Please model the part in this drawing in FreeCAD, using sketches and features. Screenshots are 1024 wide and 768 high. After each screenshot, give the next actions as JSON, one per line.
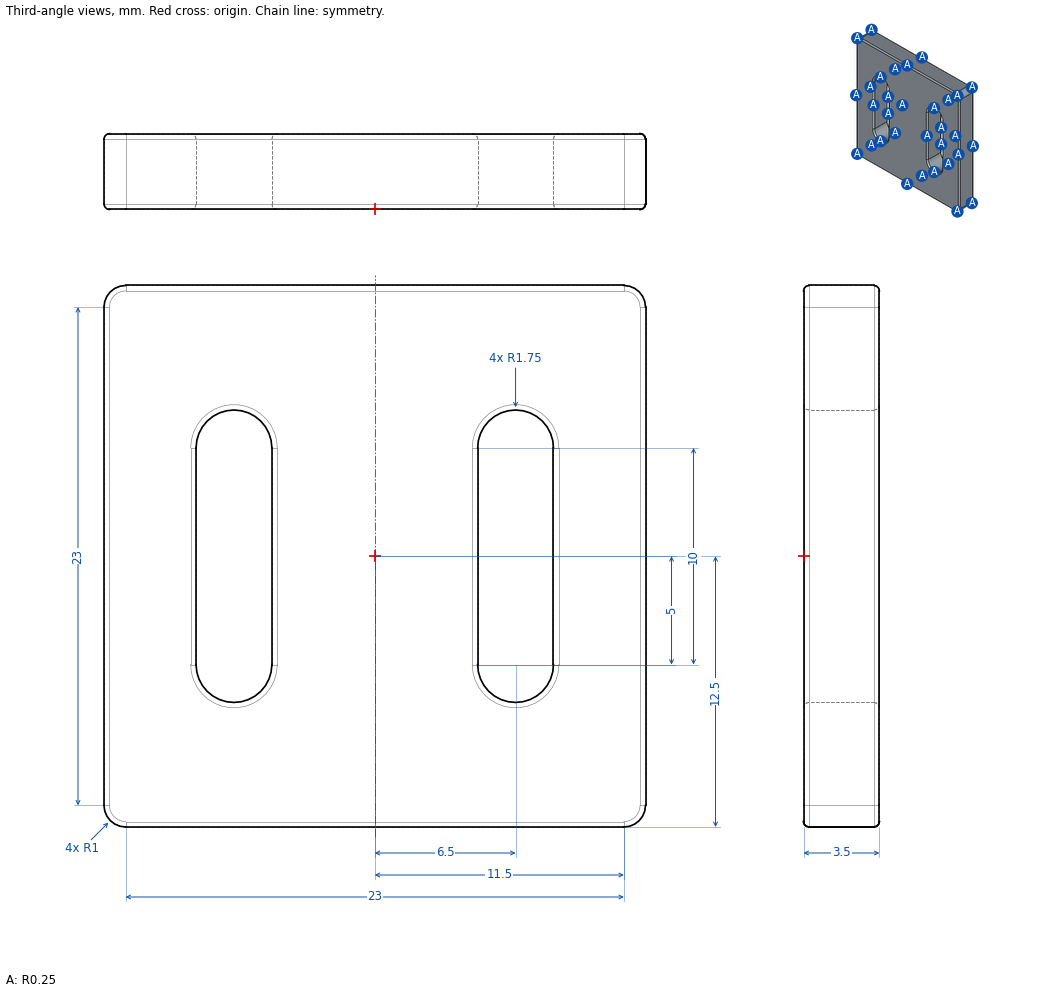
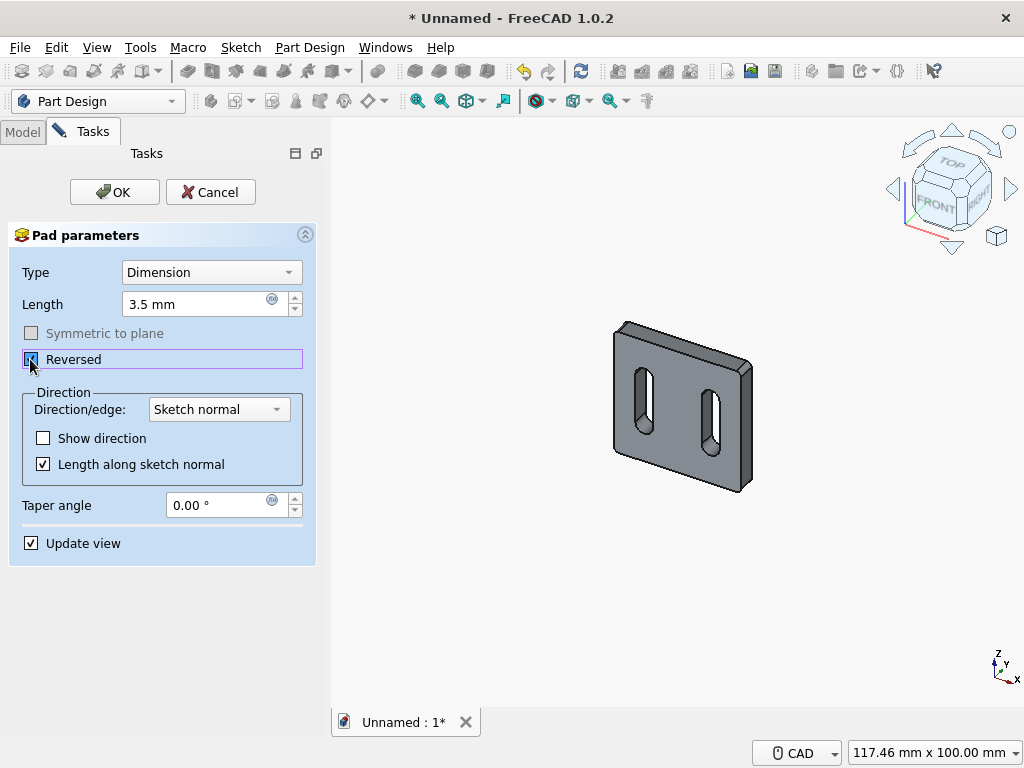
{"action": "left_click", "coordinate": [115, 192]}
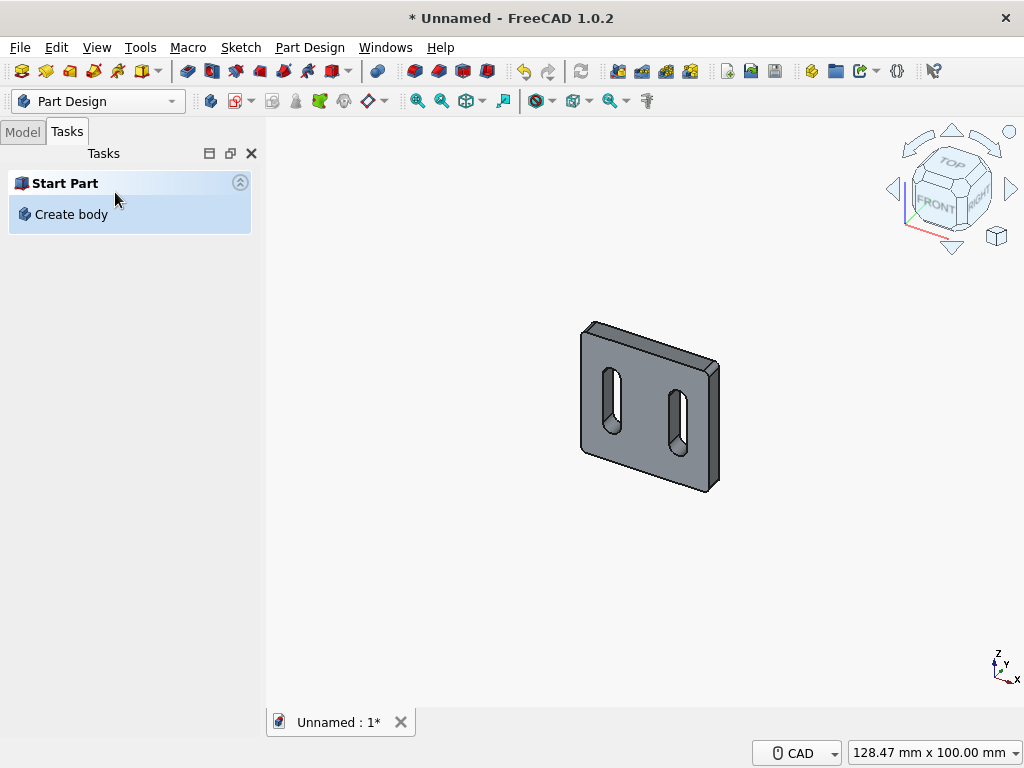
{"action": "key", "text": "v f"}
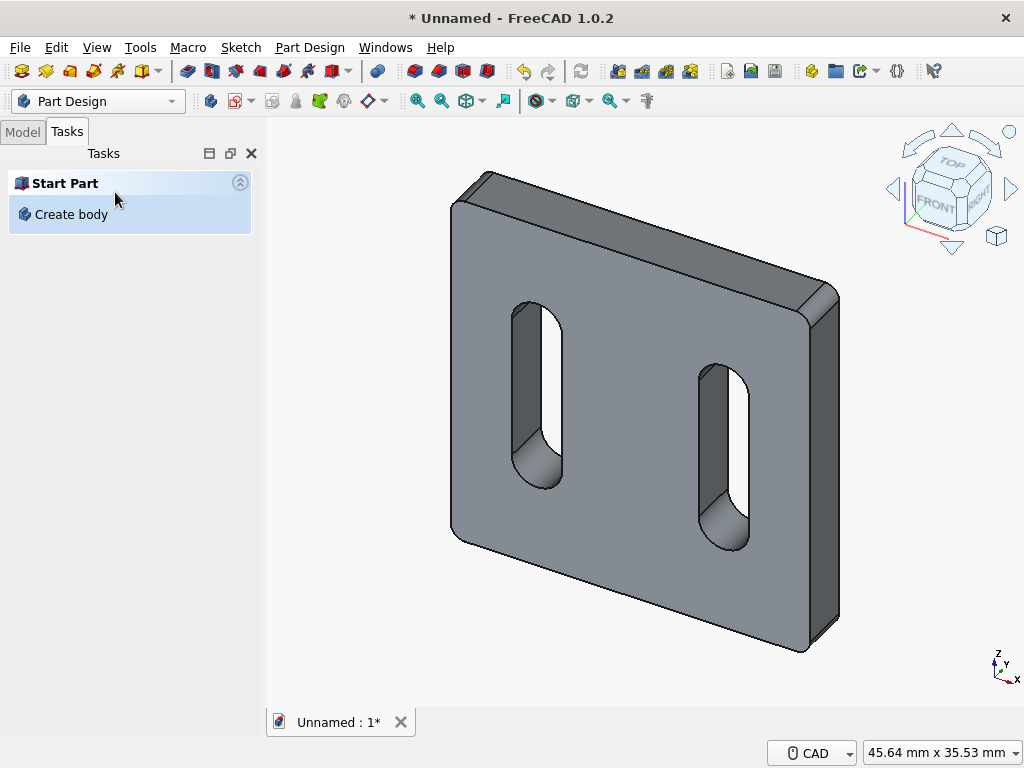
{"action": "left_click", "coordinate": [630, 328]}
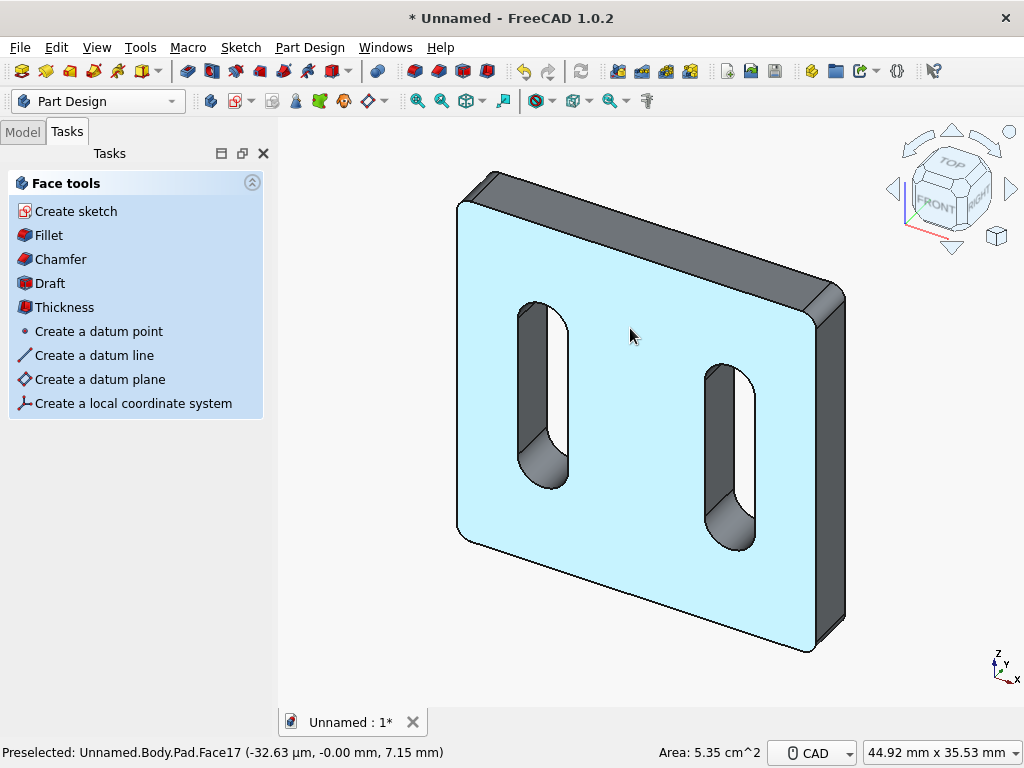
{"action": "key", "text": "0"}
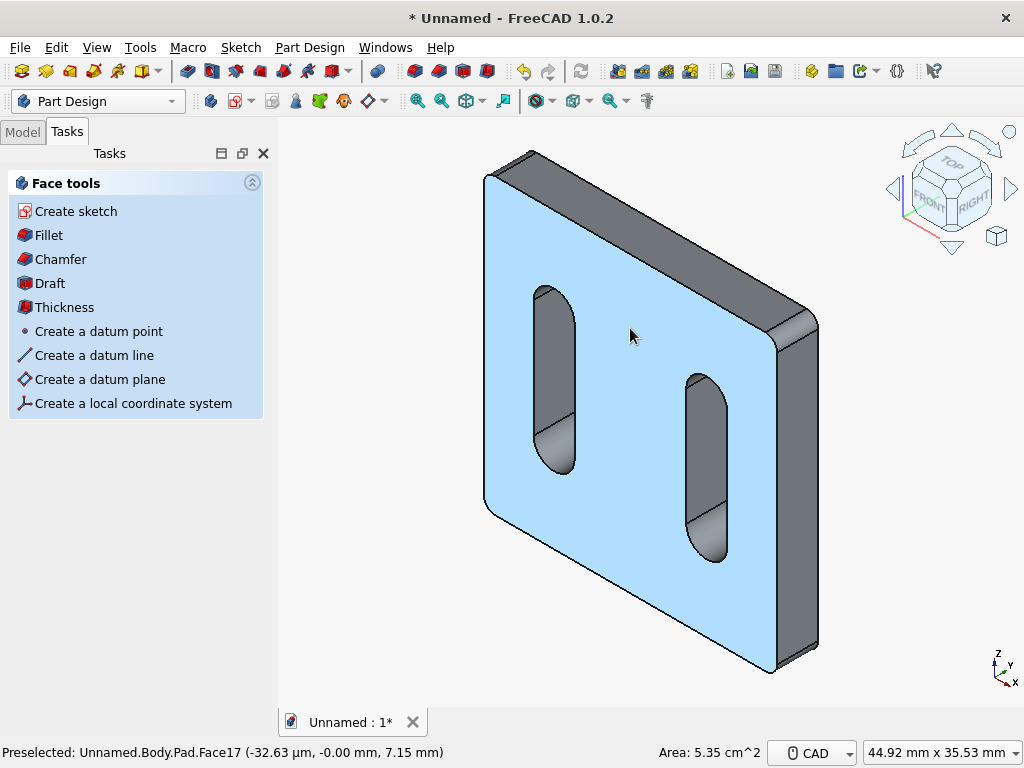
{"action": "key", "text": "2"}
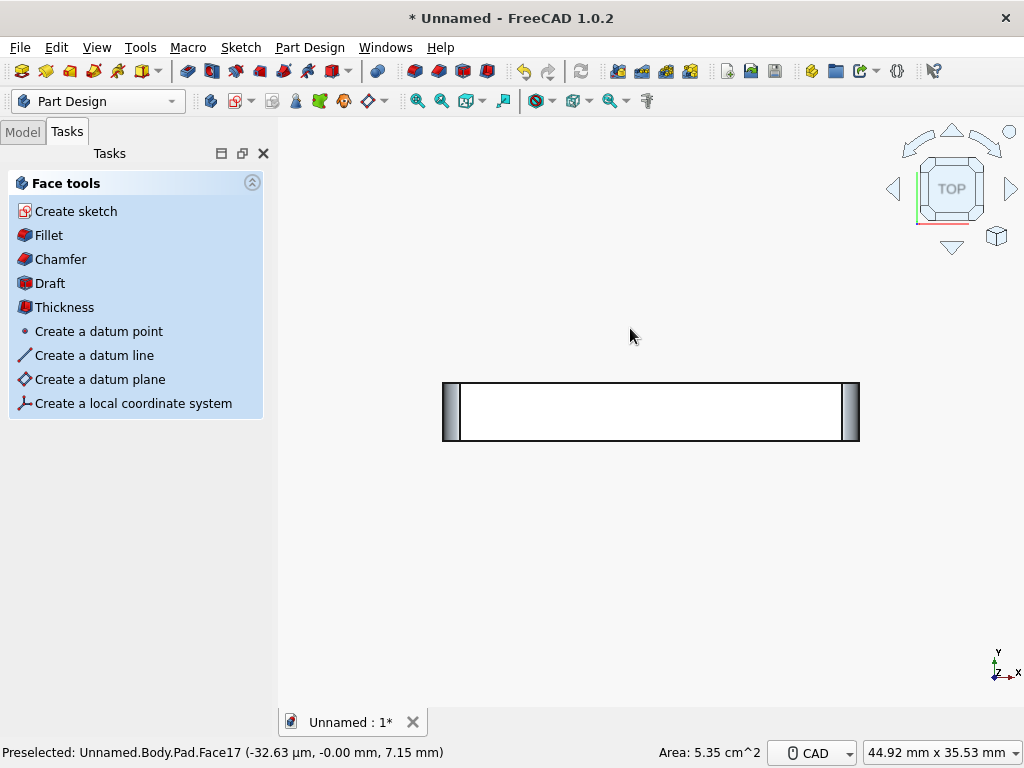
{"action": "key", "text": "1"}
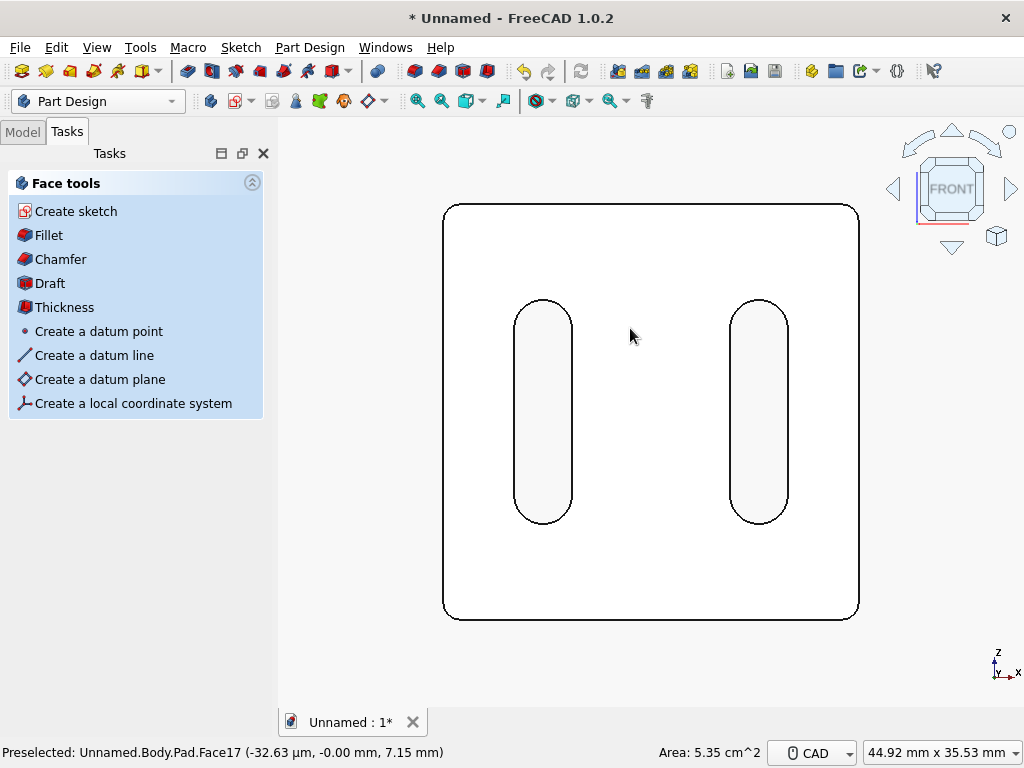
{"action": "key", "text": "3"}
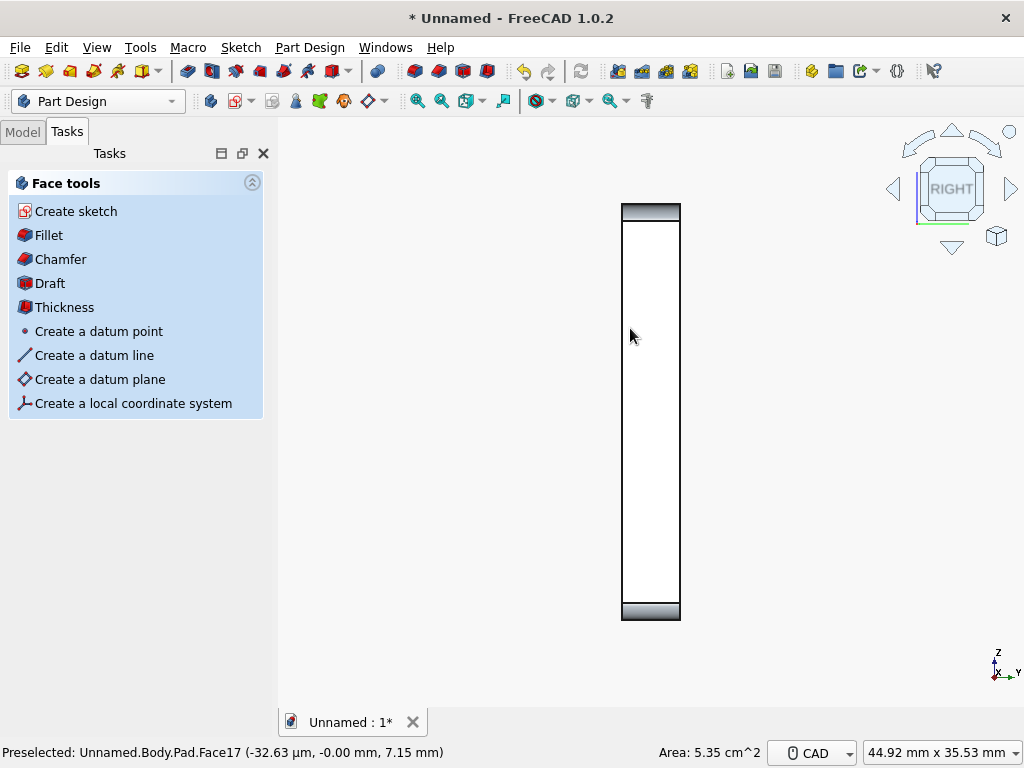
{"action": "key", "text": "5"}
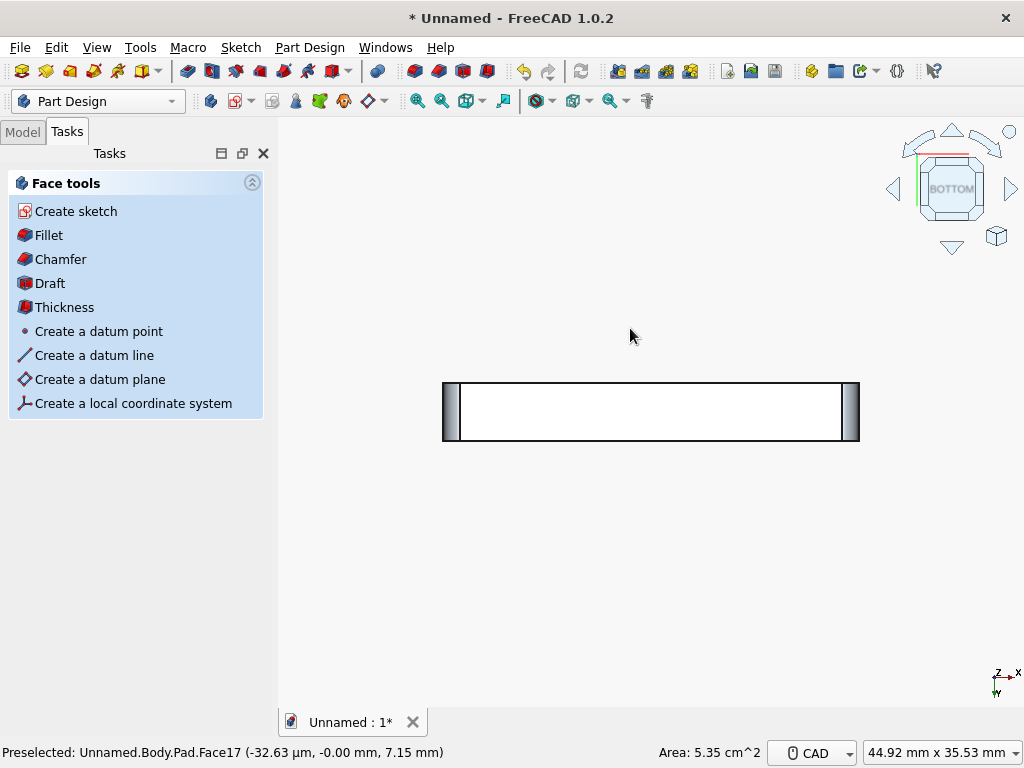
{"action": "key", "text": "4"}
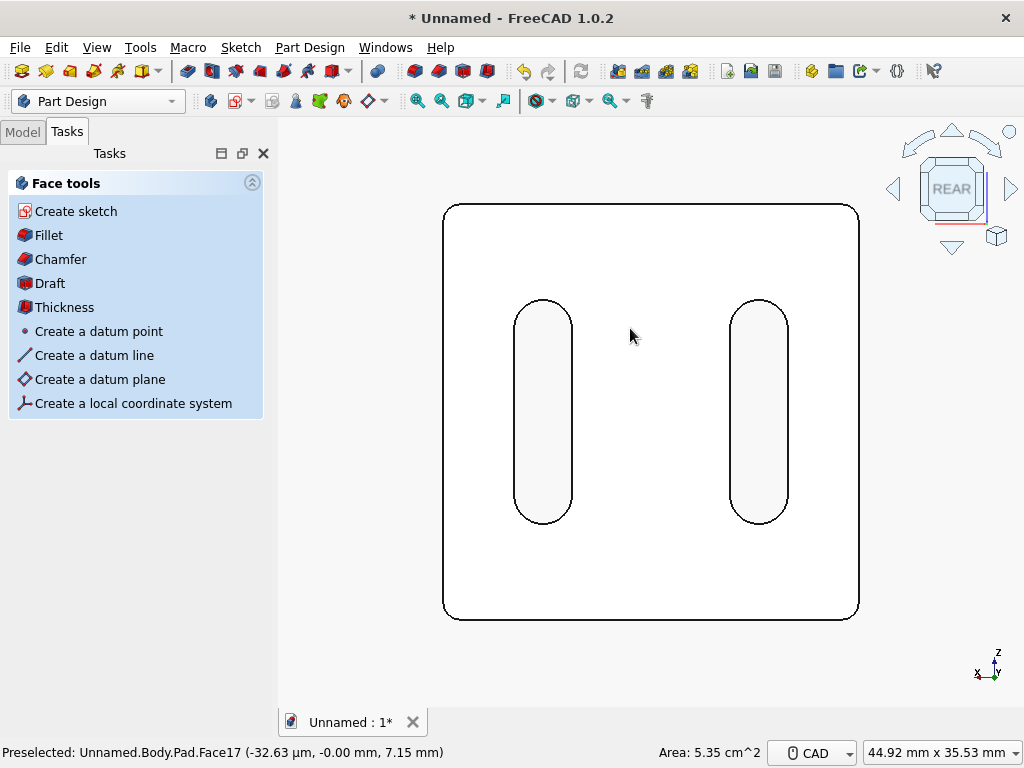
{"action": "left_click", "coordinate": [651, 292], "text": "ctrl"}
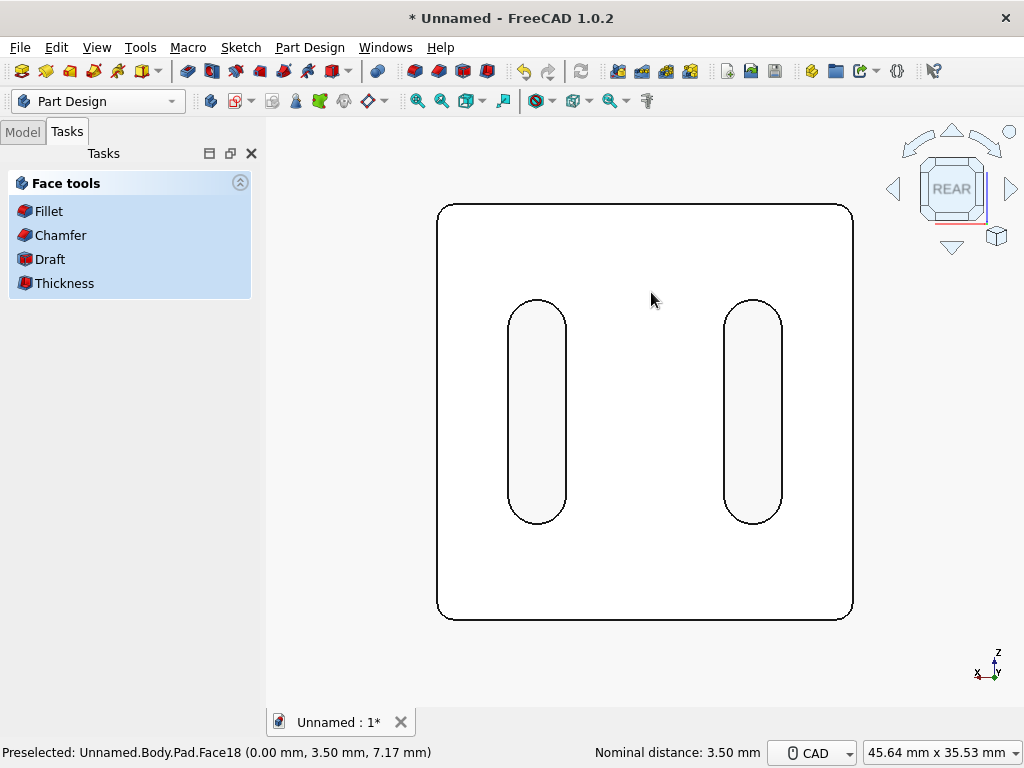
{"action": "left_click", "coordinate": [416, 72]}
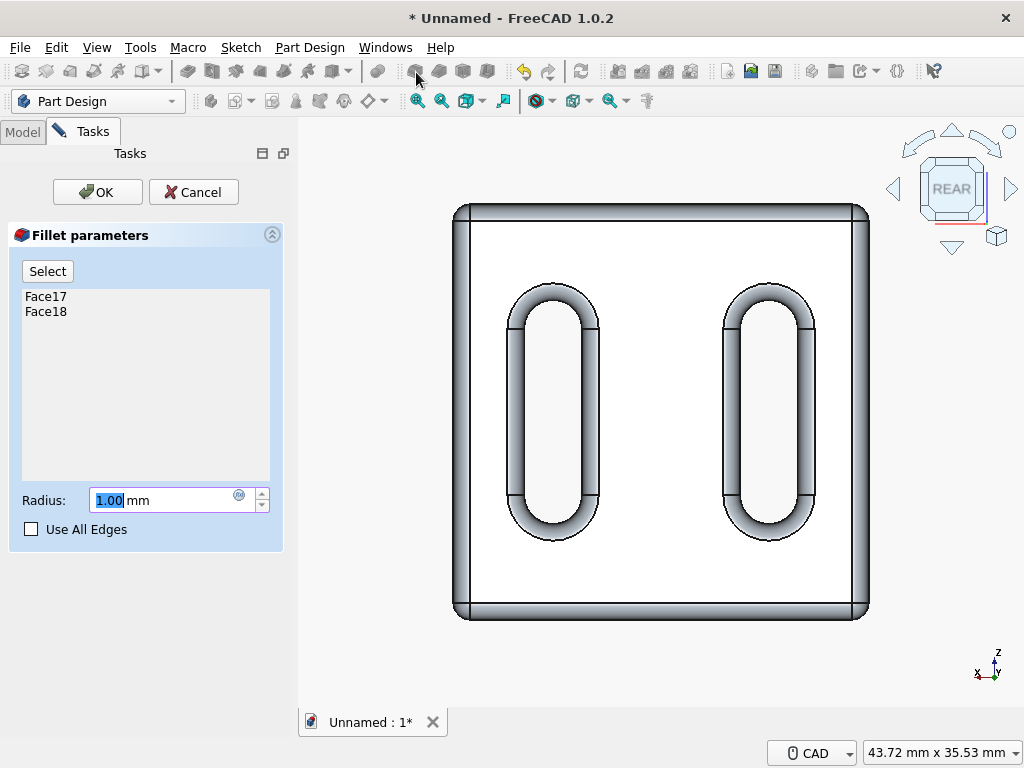
{"action": "type", "text": "0.25"}
{"action": "key", "text": "Tab"}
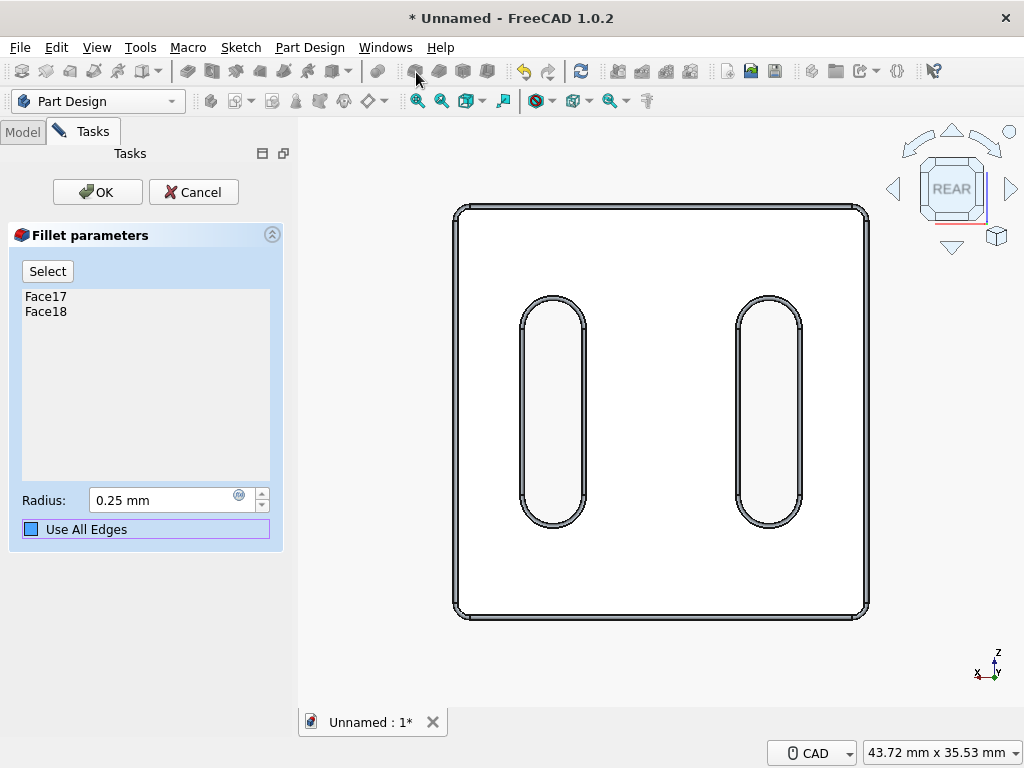
{"action": "left_click", "coordinate": [98, 192]}